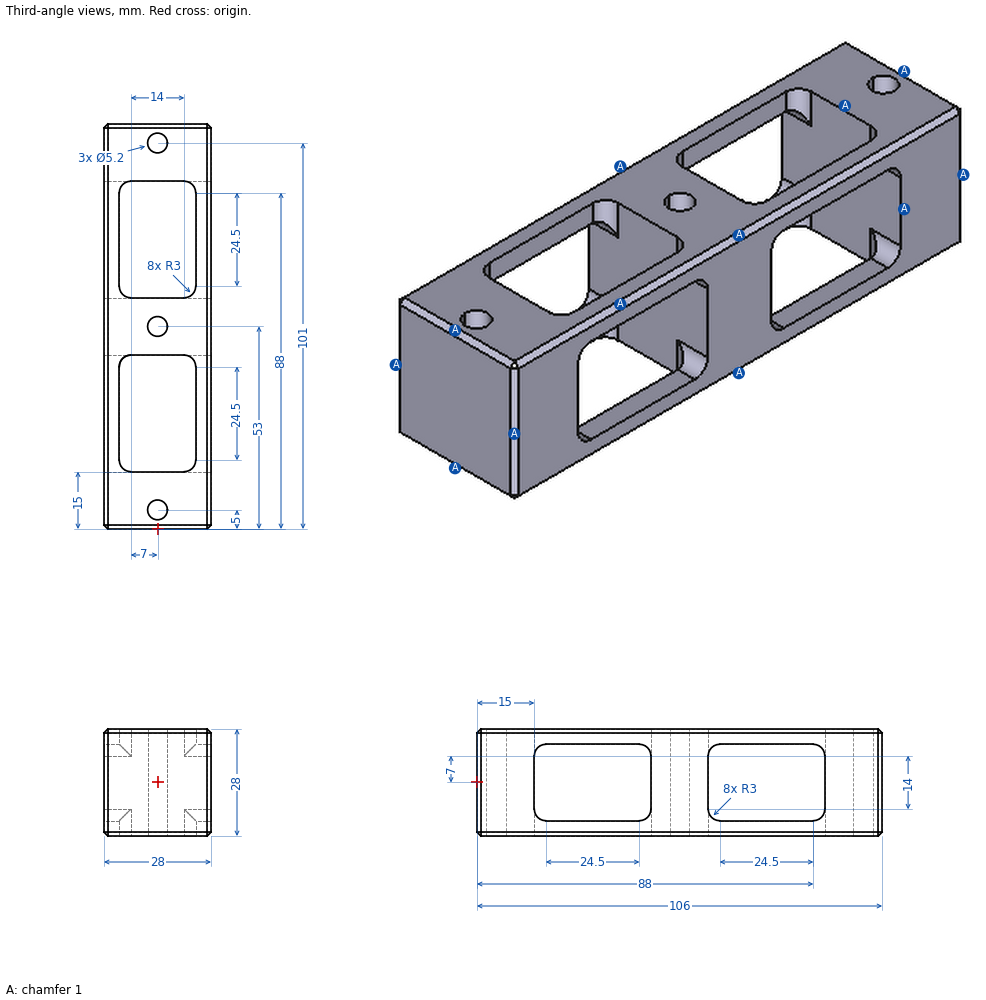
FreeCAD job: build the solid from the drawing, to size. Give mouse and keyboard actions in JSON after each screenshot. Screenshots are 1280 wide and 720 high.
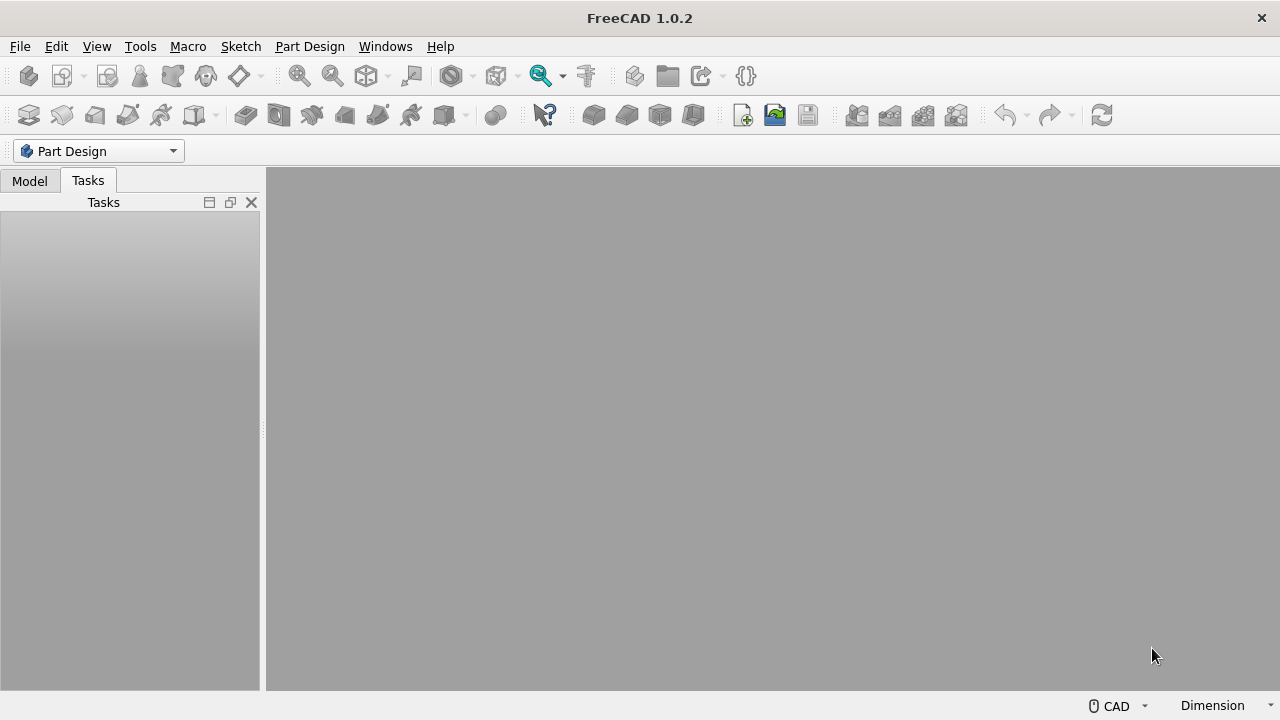
{"action": "left_click", "coordinate": [742, 116]}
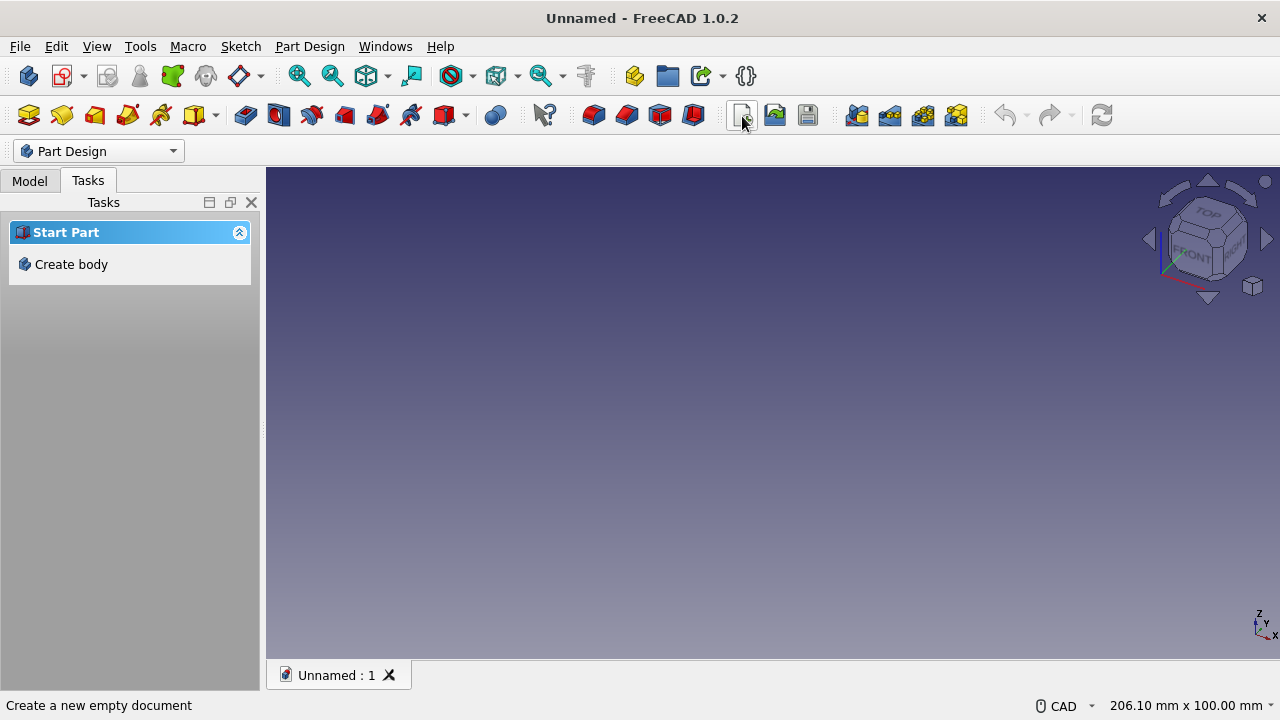
{"action": "left_click", "coordinate": [62, 76]}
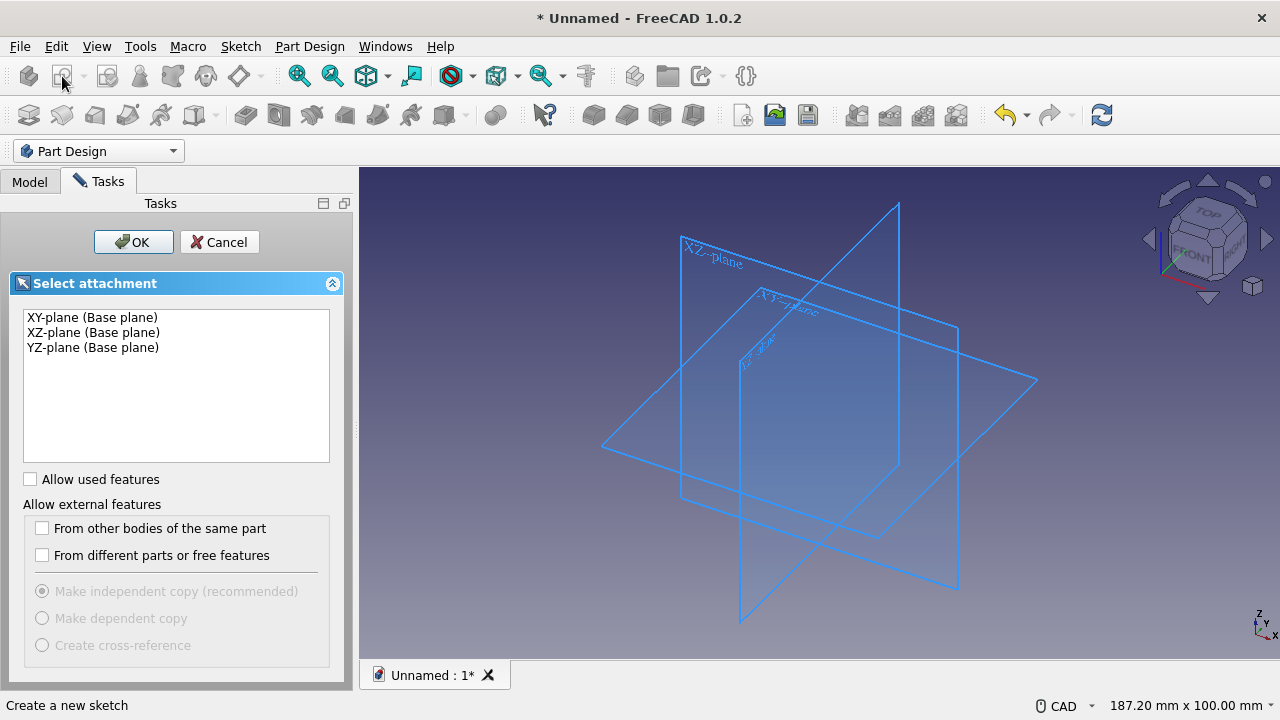
{"action": "left_click", "coordinate": [84, 332]}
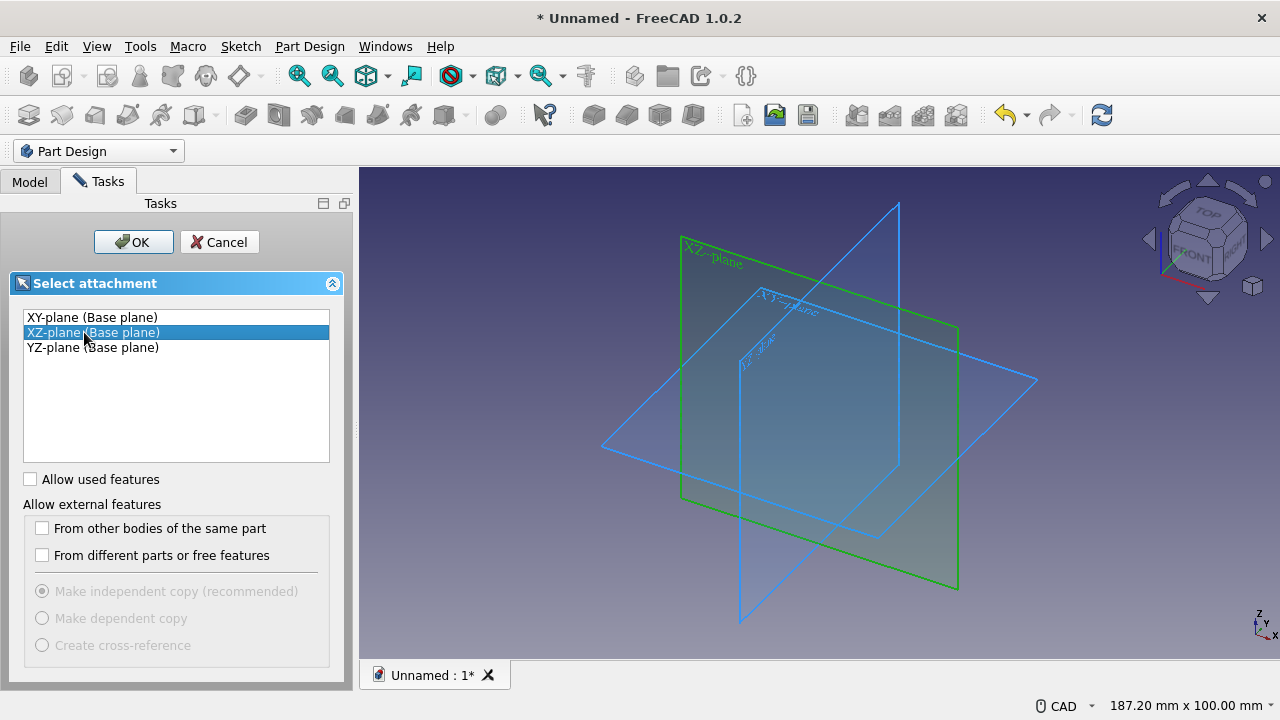
{"action": "left_click", "coordinate": [134, 242]}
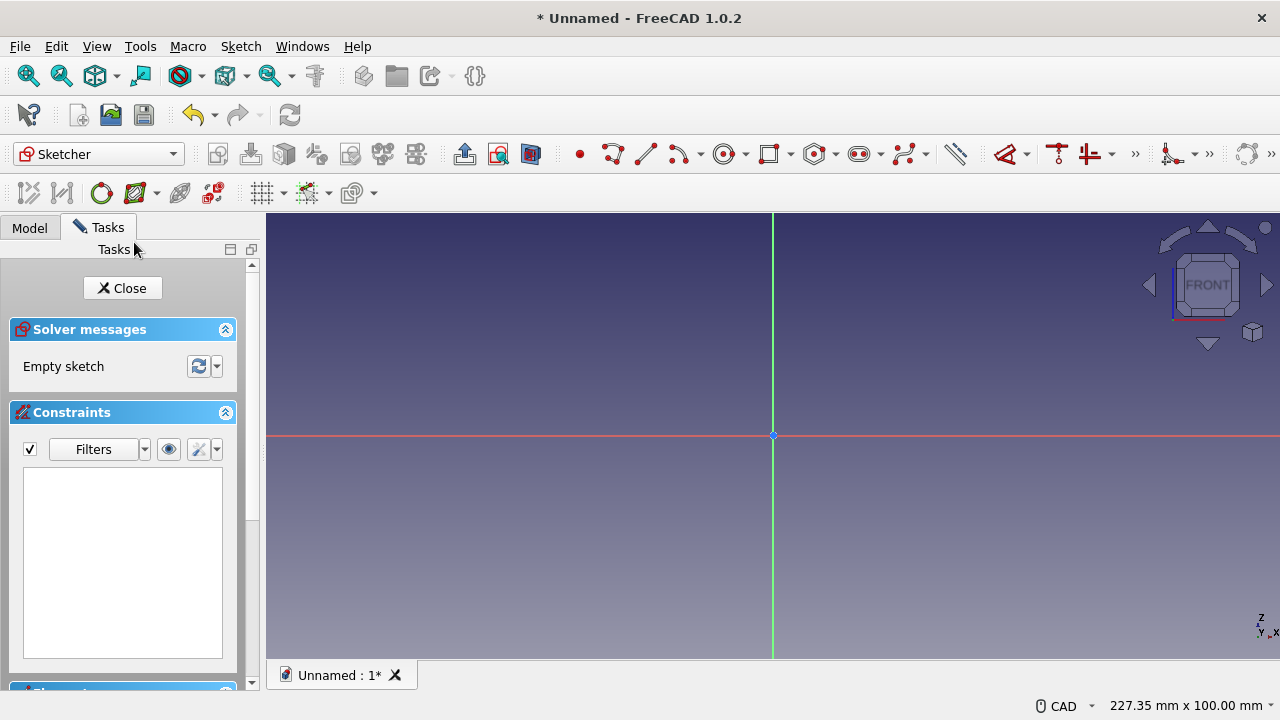
{"action": "scroll", "coordinate": [829, 436], "scroll_direction": "up", "scroll_amount": 4}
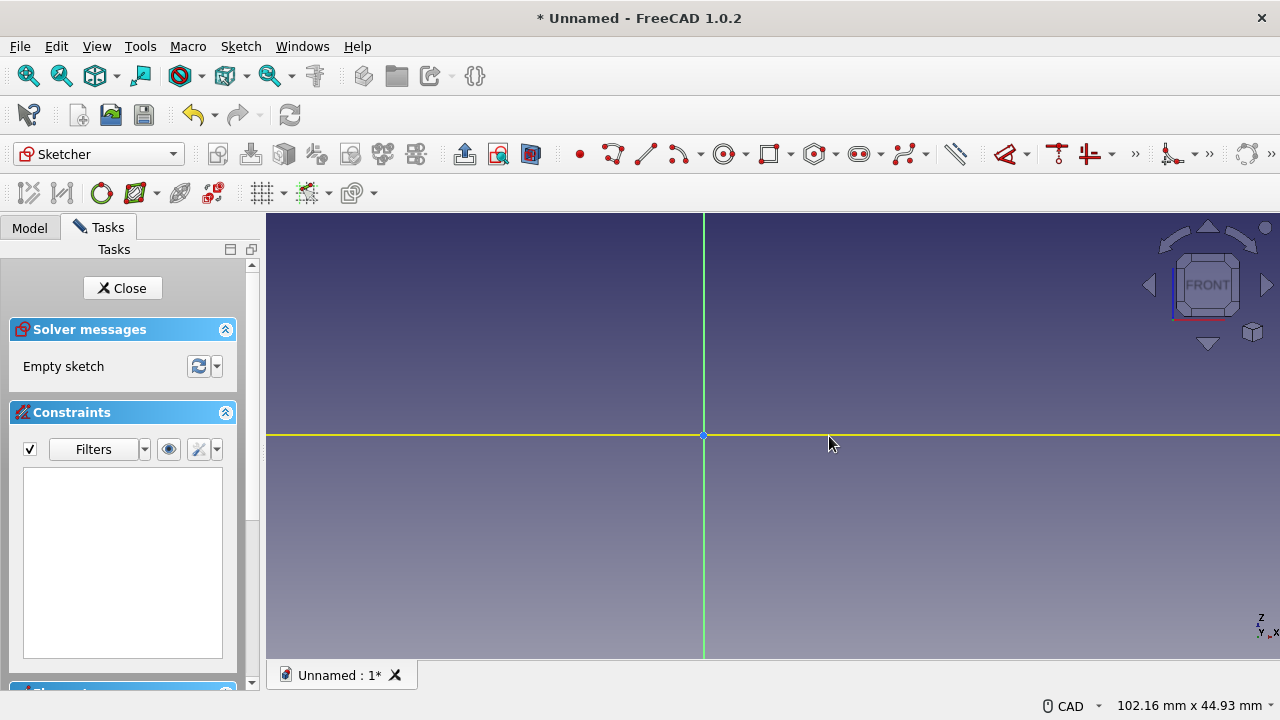
{"action": "key", "text": "g v"}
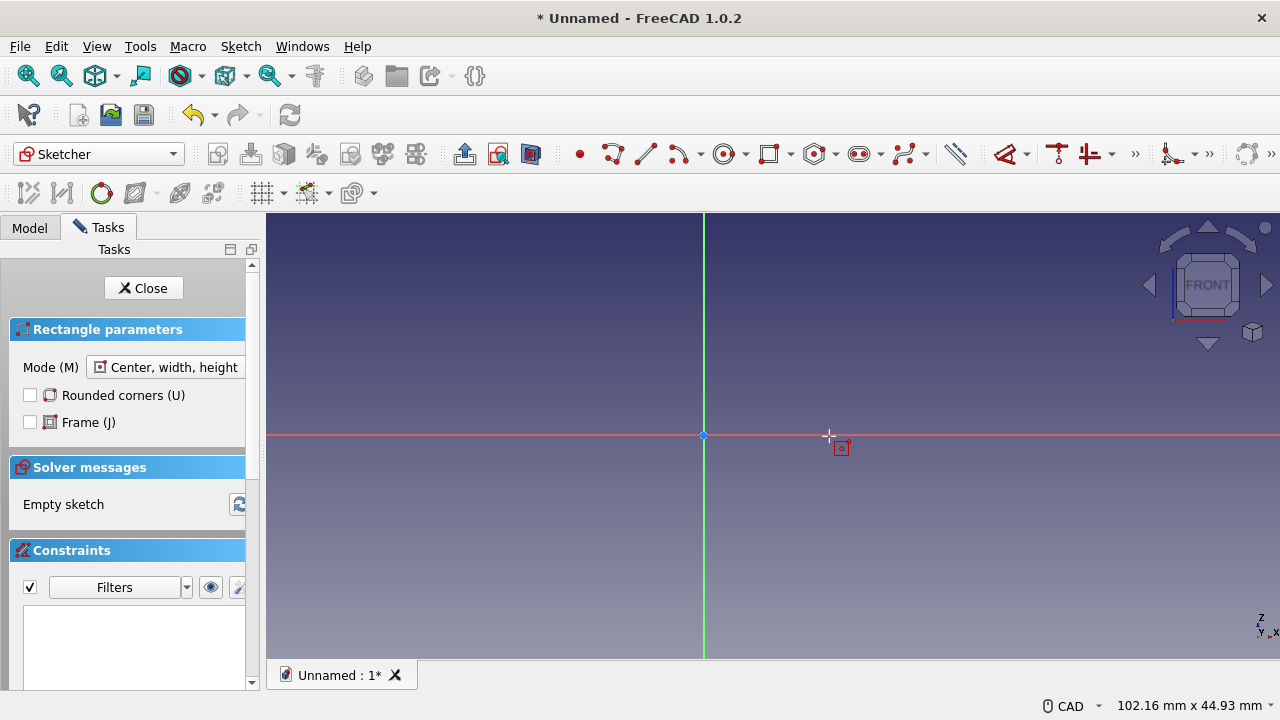
{"action": "left_click", "coordinate": [704, 435]}
{"action": "mouse_move", "coordinate": [843, 296]}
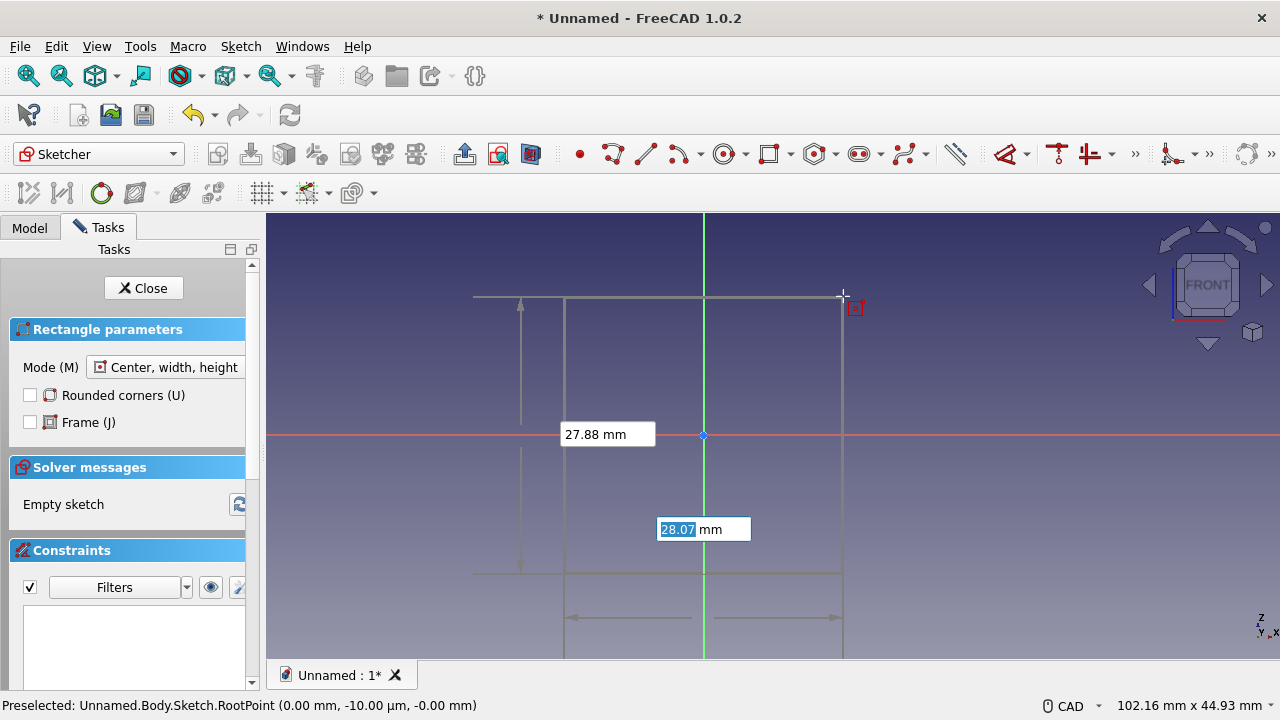
{"action": "type", "text": "28"}
{"action": "key", "text": "Tab"}
{"action": "type", "text": "28"}
{"action": "key", "text": "Return"}
{"action": "key", "text": "Escape"}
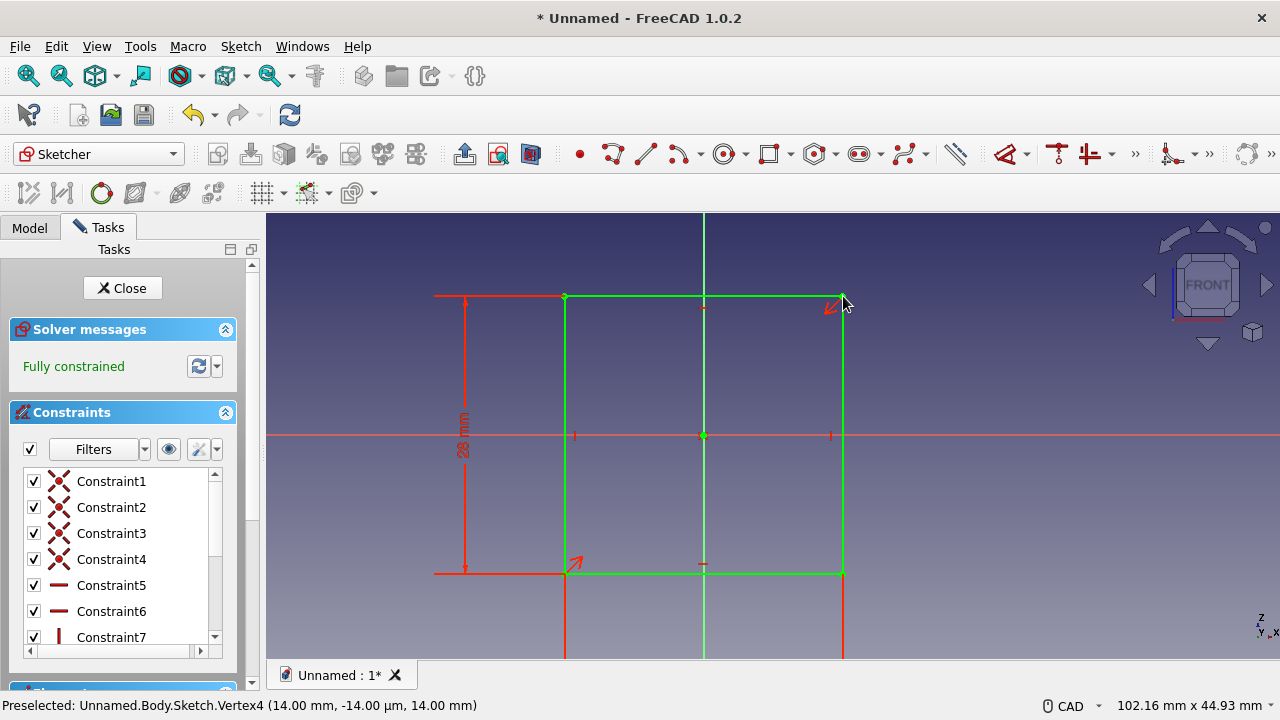
{"action": "left_click", "coordinate": [123, 288]}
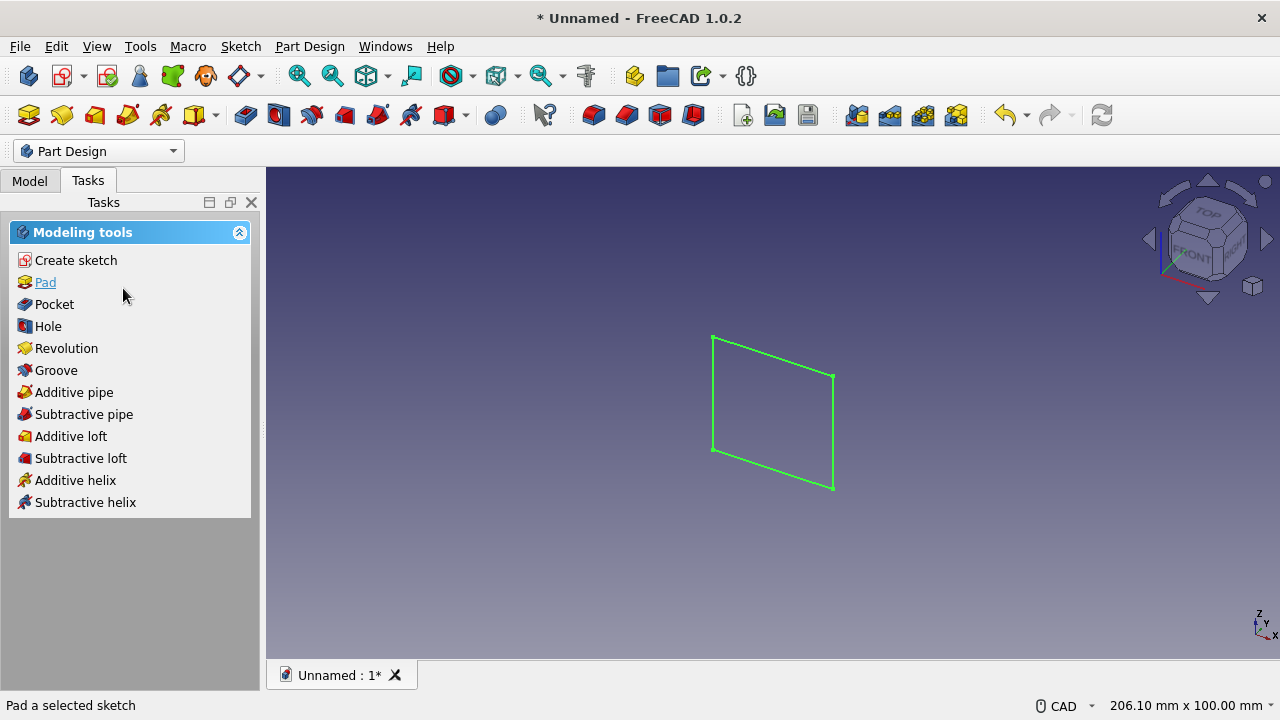
{"action": "left_click", "coordinate": [29, 116]}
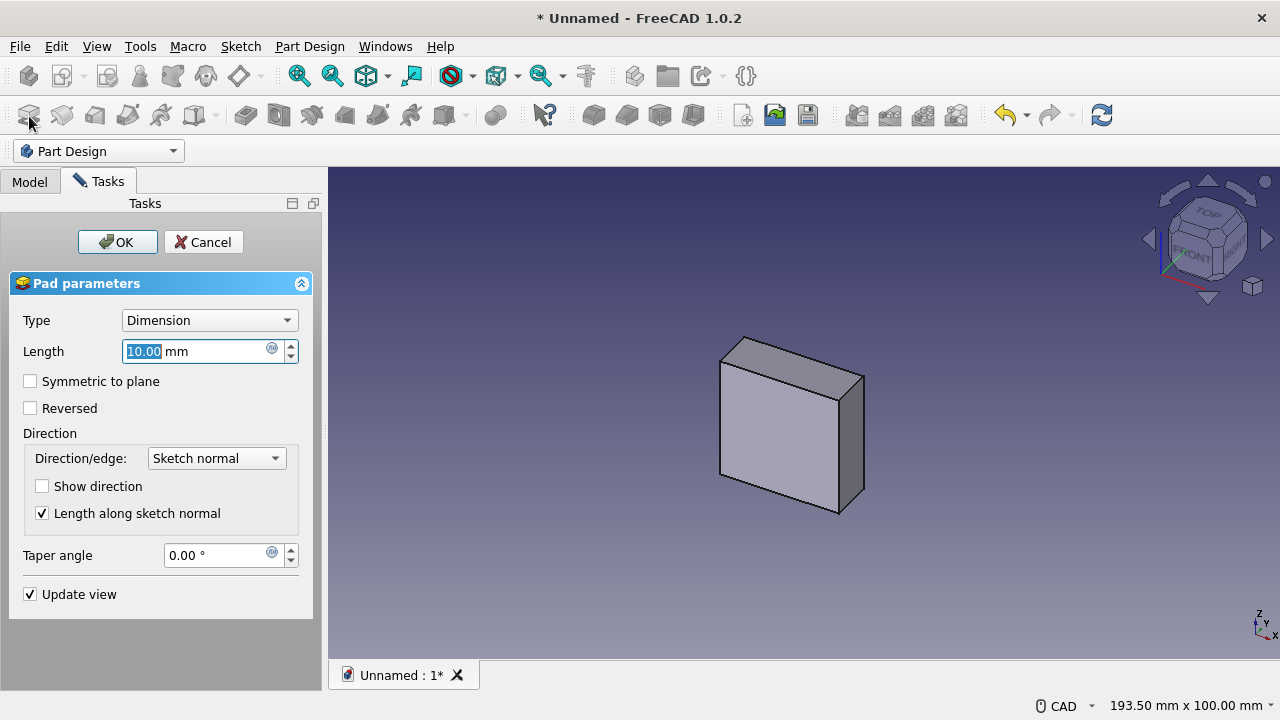
{"action": "type", "text": "106"}
{"action": "key", "text": "Tab"}